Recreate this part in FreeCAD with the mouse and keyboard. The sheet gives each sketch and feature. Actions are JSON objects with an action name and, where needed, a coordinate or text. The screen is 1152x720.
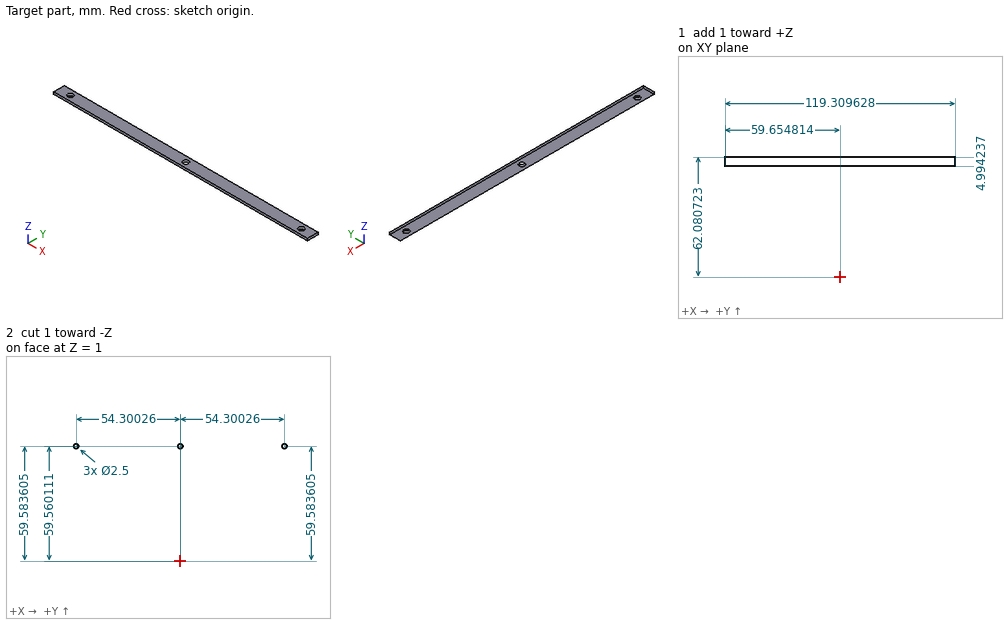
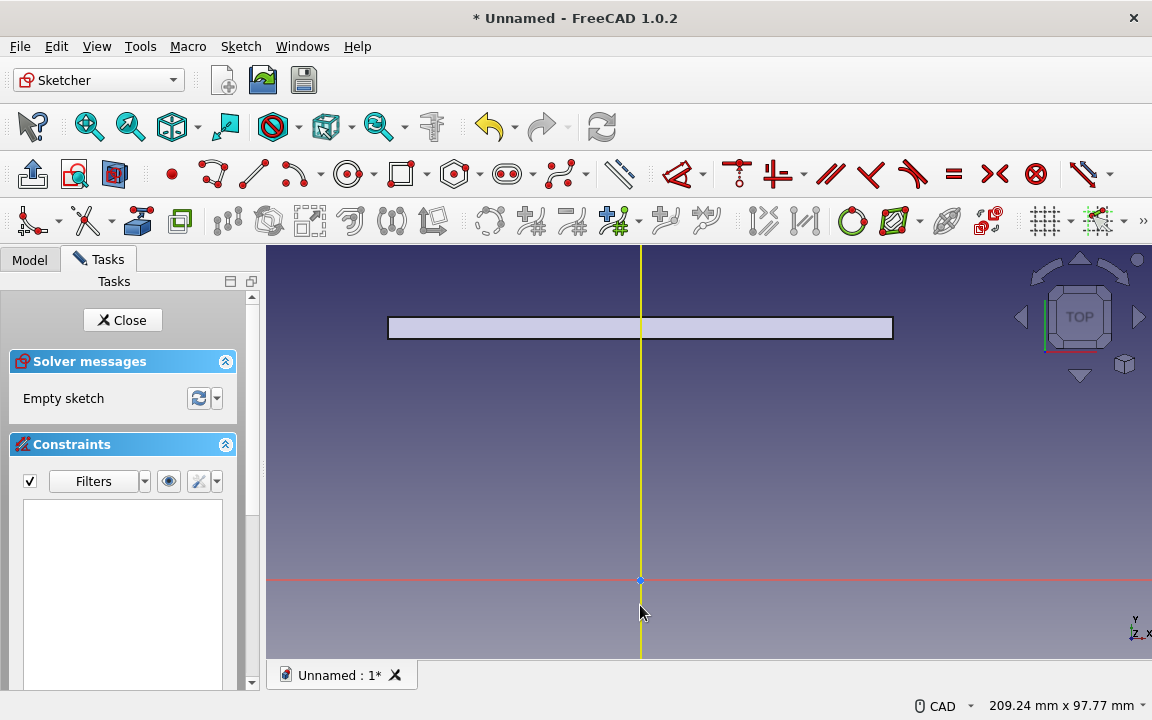
{"action": "key", "text": "g c"}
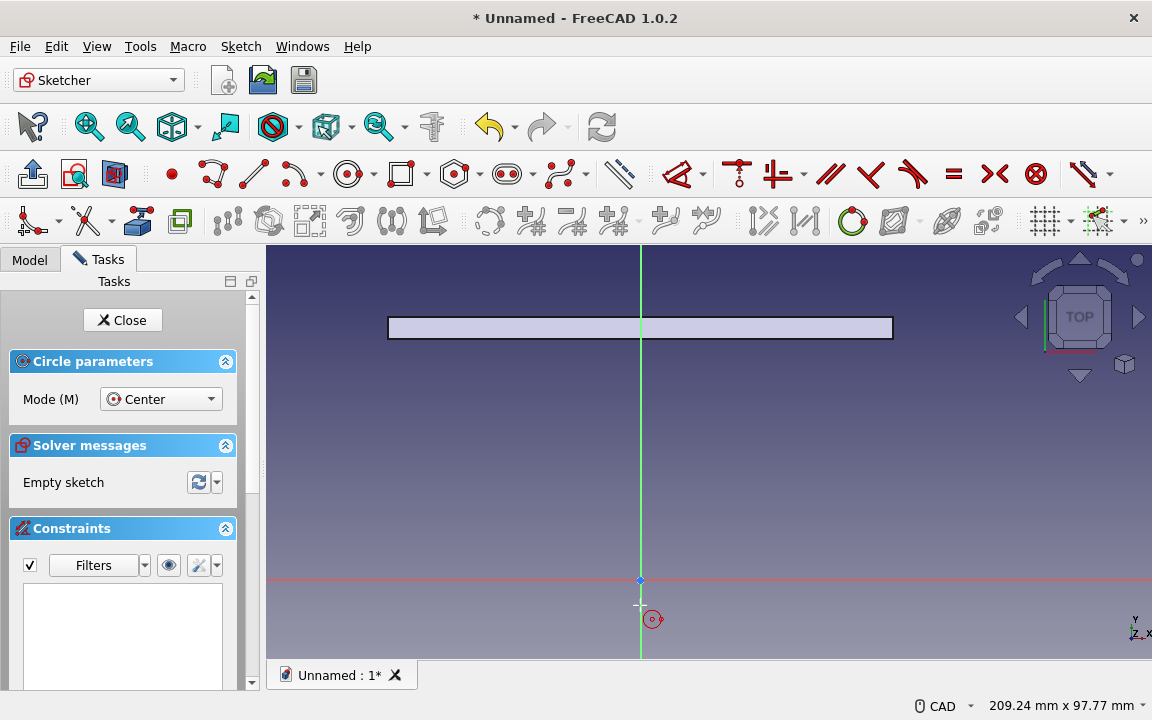
{"action": "scroll", "coordinate": [411, 328], "scroll_direction": "up", "scroll_amount": 8}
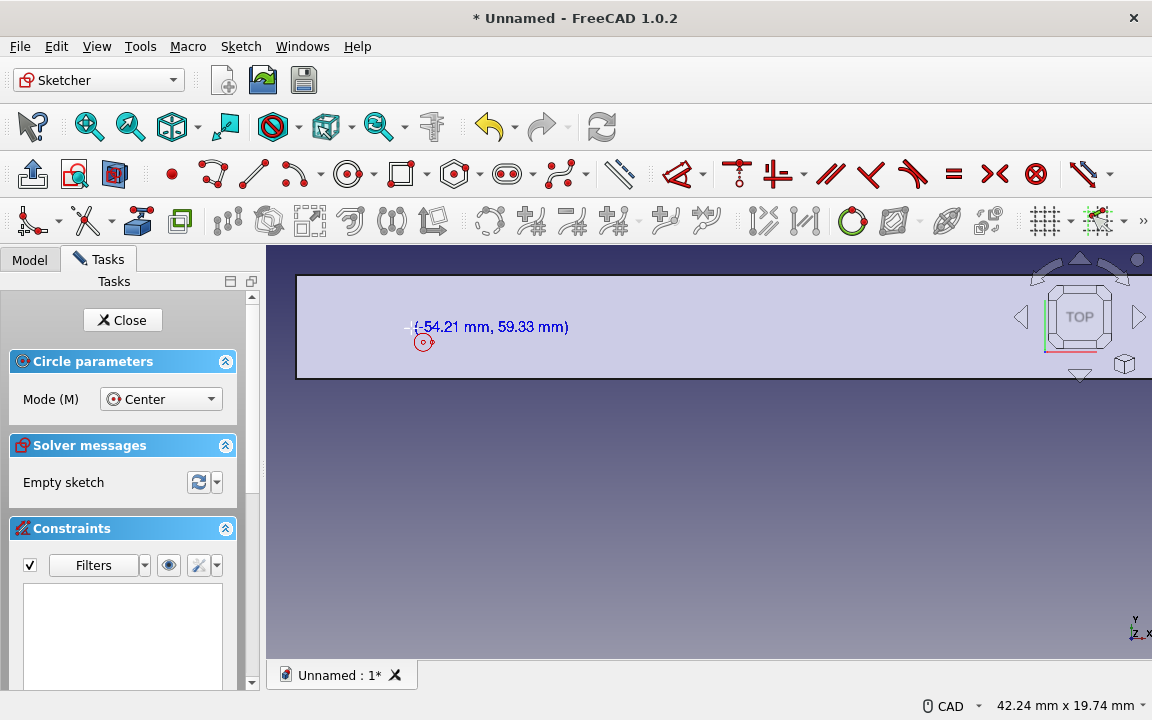
{"action": "scroll", "coordinate": [411, 329], "scroll_direction": "down", "scroll_amount": 8}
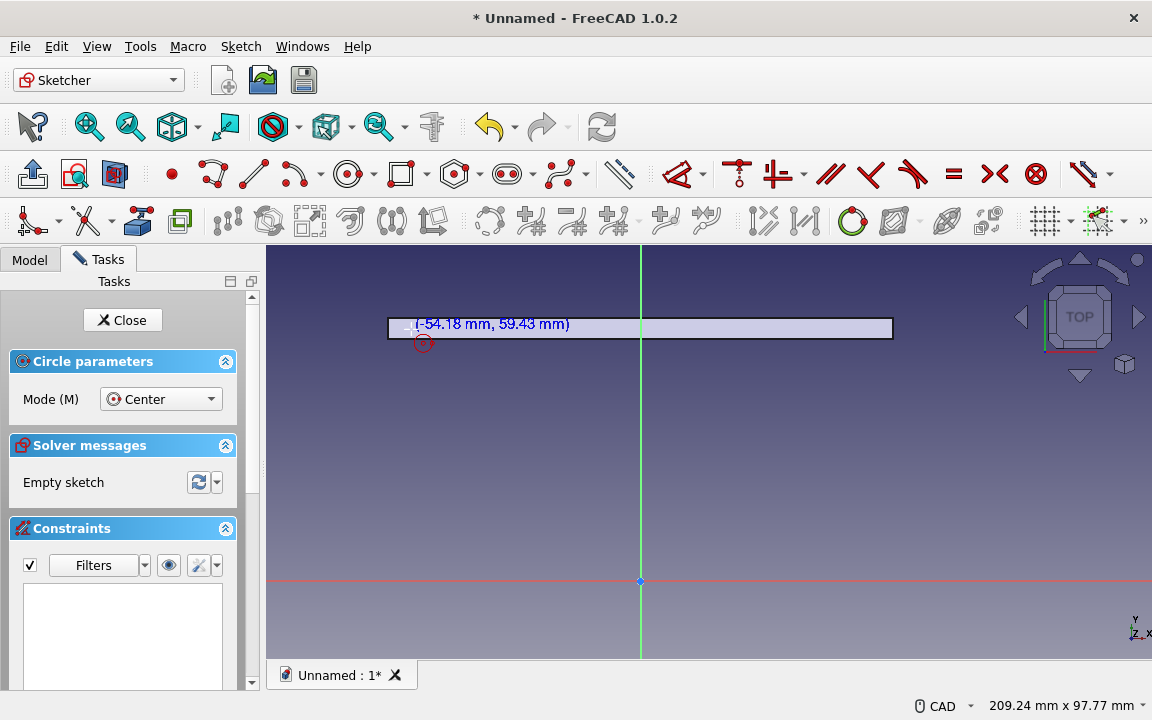
{"action": "left_click", "coordinate": [411, 329]}
{"action": "mouse_move", "coordinate": [414, 325]}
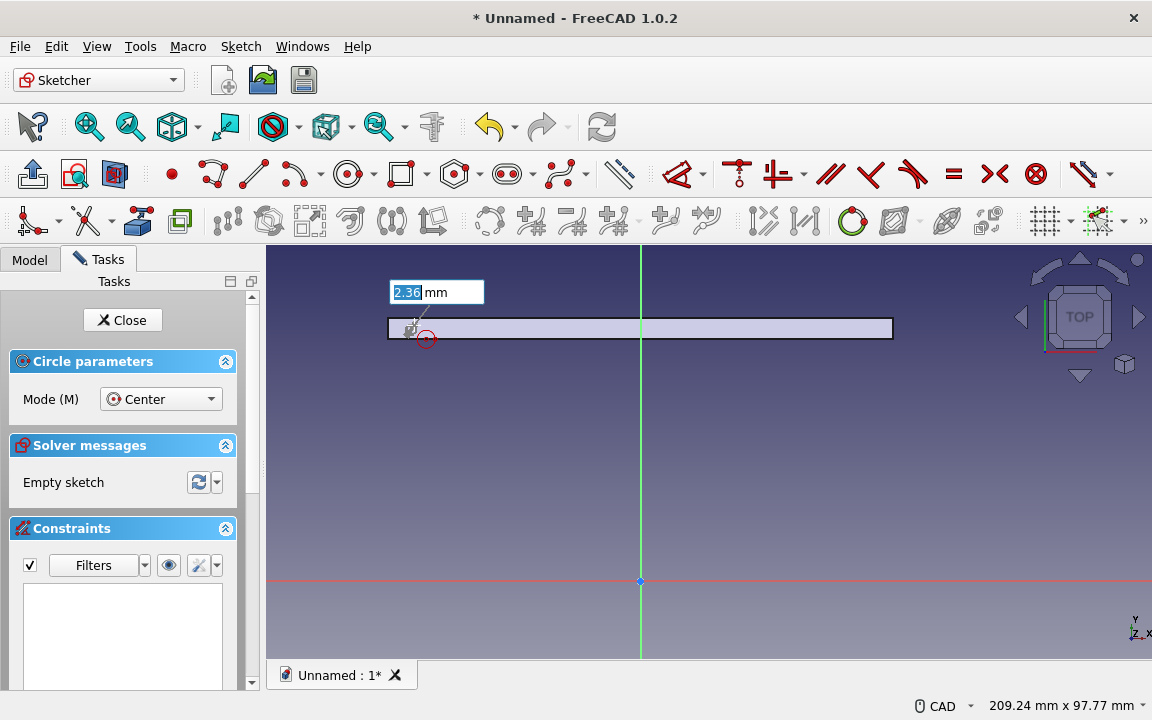
{"action": "type", "text": "2.5"}
{"action": "key", "text": "Return"}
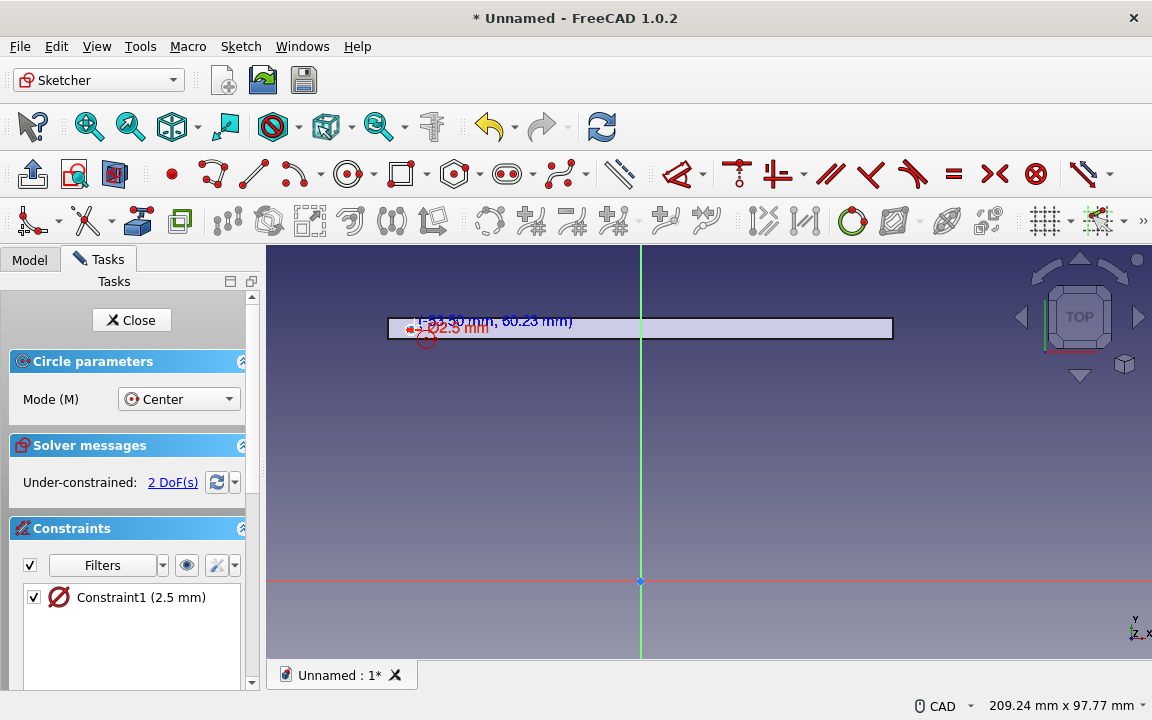
{"action": "scroll", "coordinate": [641, 329], "scroll_direction": "up", "scroll_amount": 8}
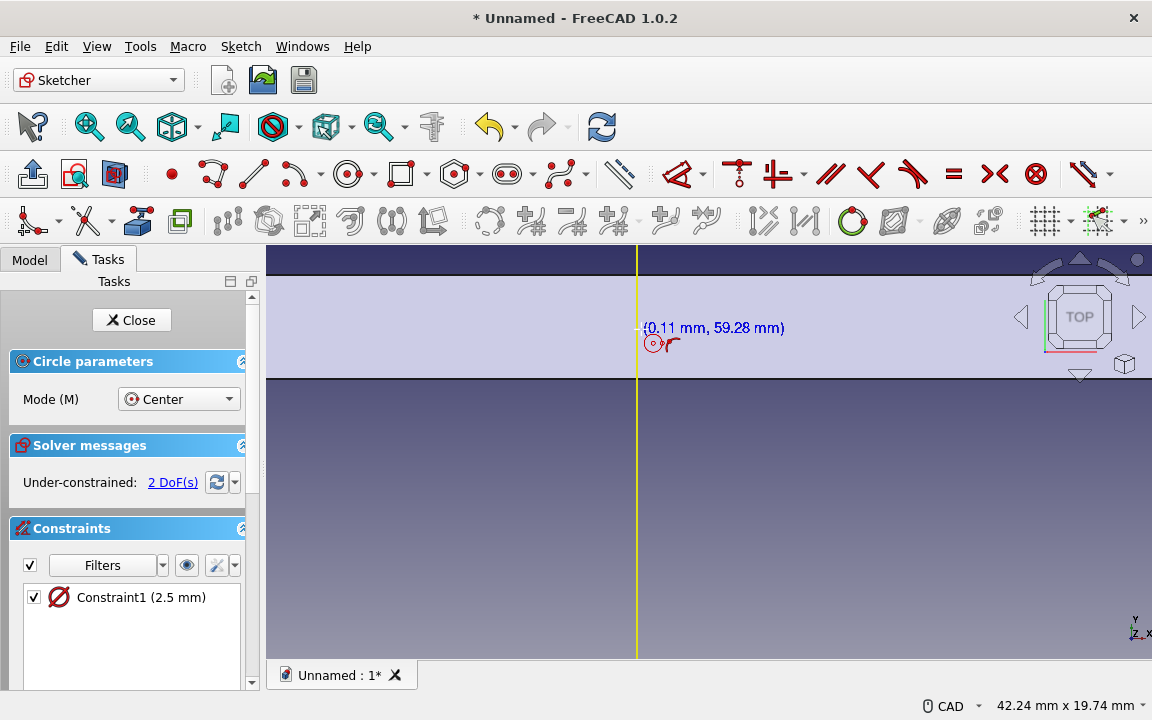
{"action": "scroll", "coordinate": [641, 329], "scroll_direction": "down", "scroll_amount": 8}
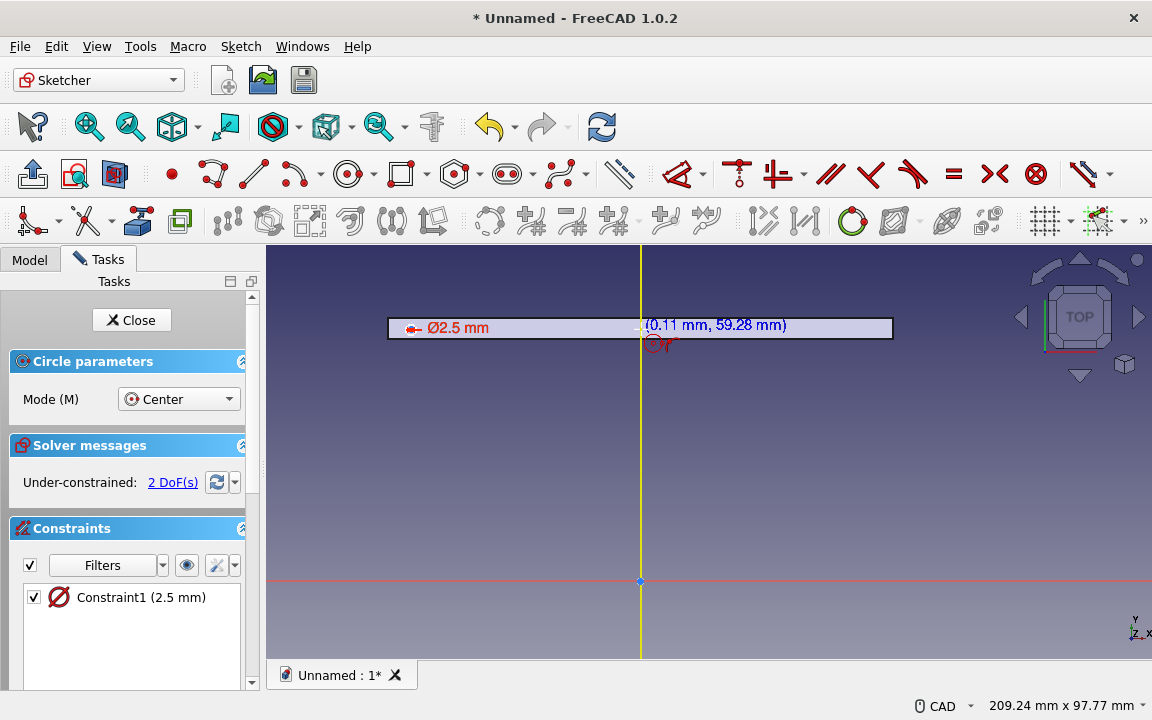
{"action": "left_click", "coordinate": [641, 329]}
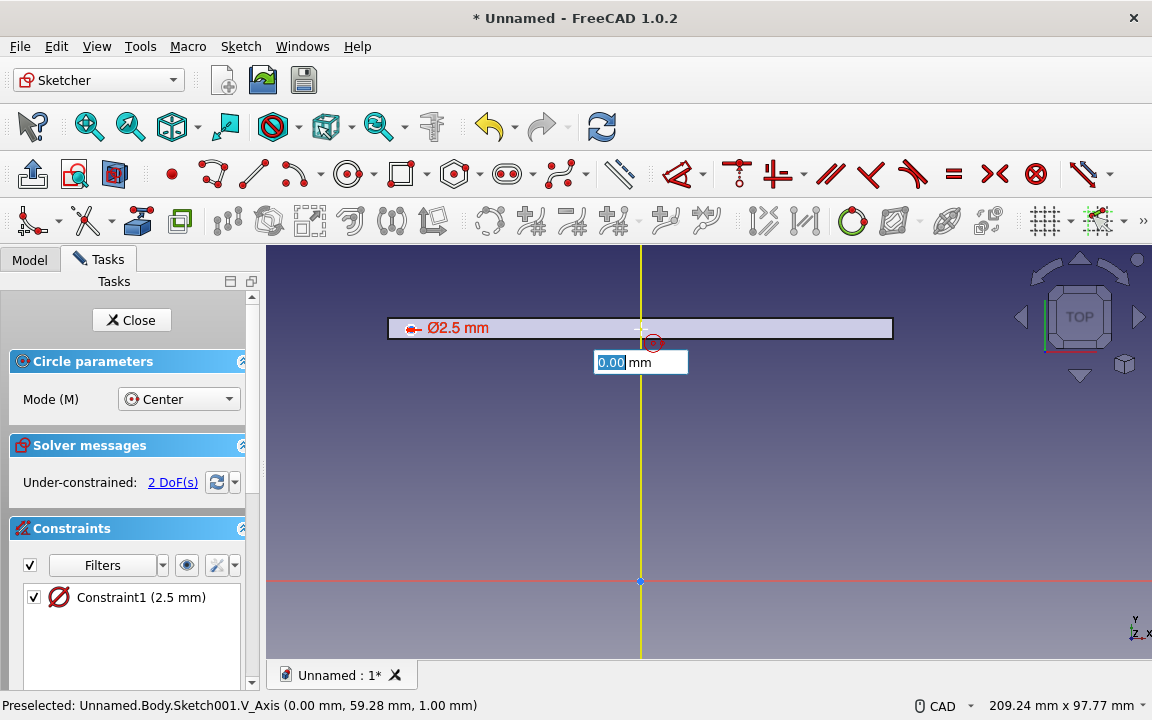
{"action": "scroll", "coordinate": [646, 327], "scroll_direction": "up", "scroll_amount": 6}
{"action": "mouse_move", "coordinate": [643, 327]}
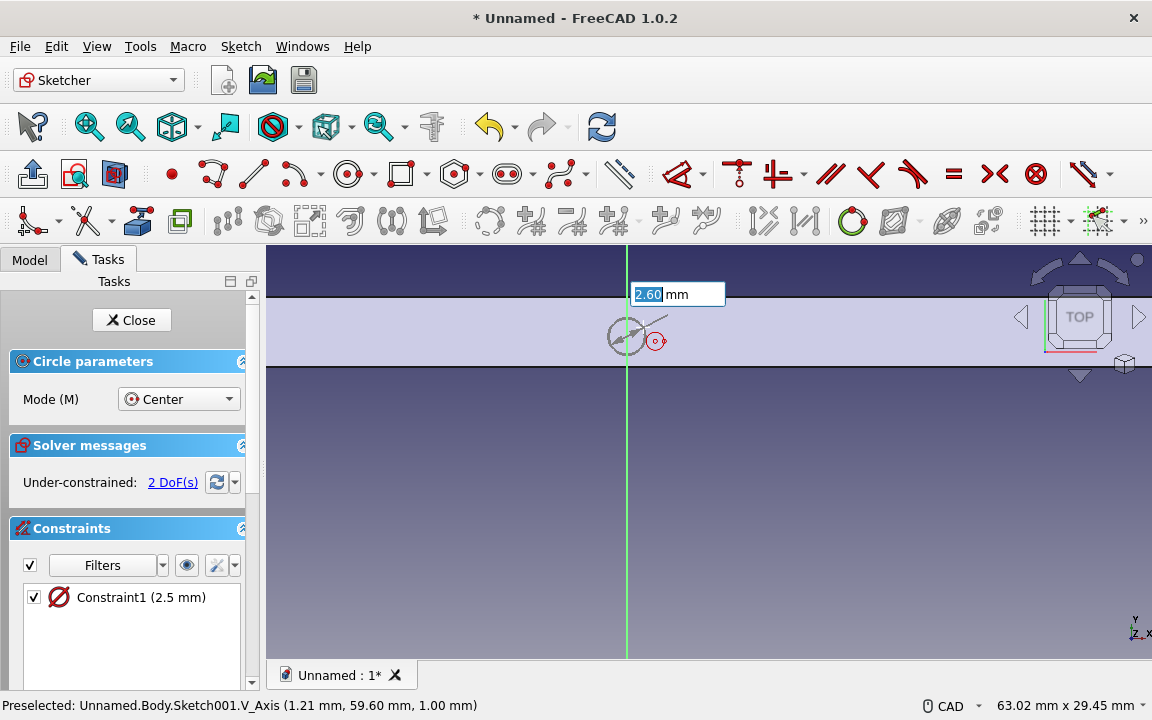
{"action": "type", "text": "2.5"}
{"action": "key", "text": "Return"}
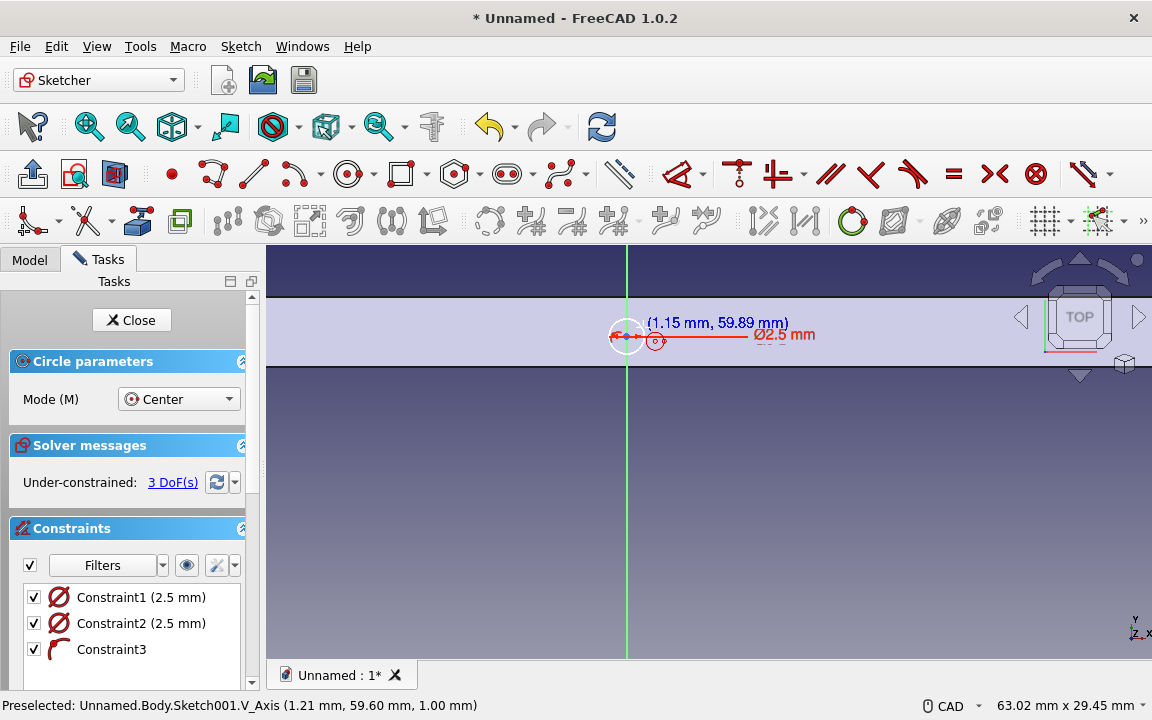
{"action": "scroll", "coordinate": [646, 327], "scroll_direction": "down", "scroll_amount": 6}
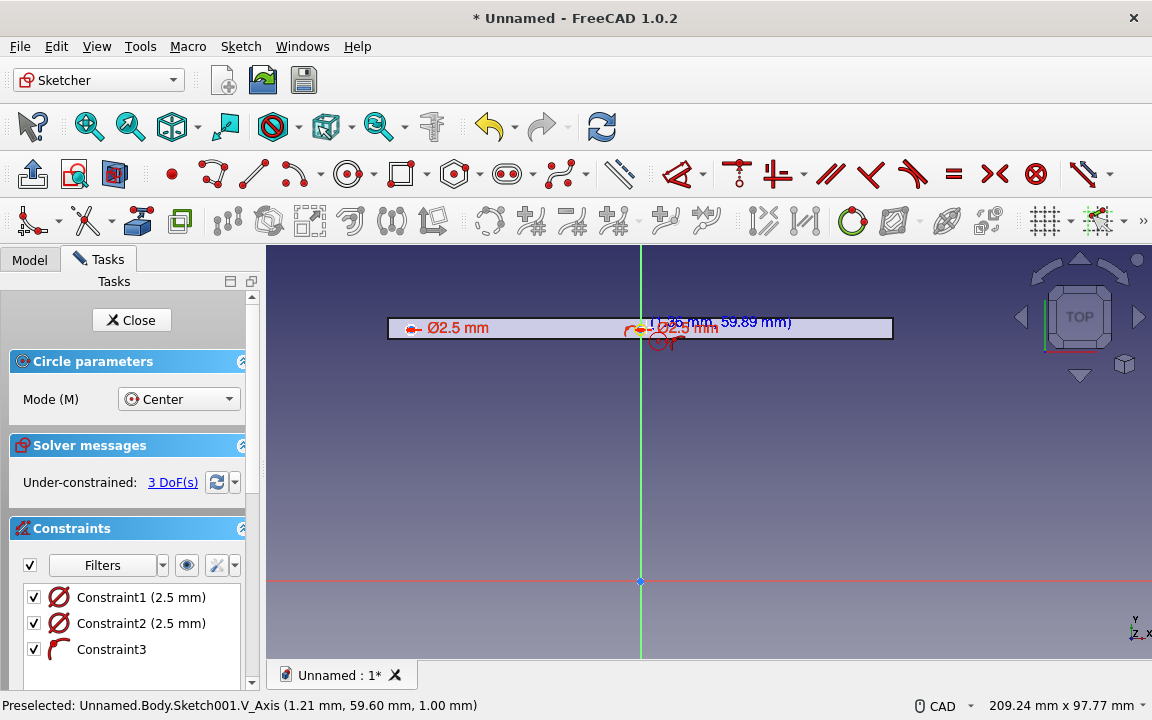
{"action": "scroll", "coordinate": [870, 329], "scroll_direction": "up", "scroll_amount": 8}